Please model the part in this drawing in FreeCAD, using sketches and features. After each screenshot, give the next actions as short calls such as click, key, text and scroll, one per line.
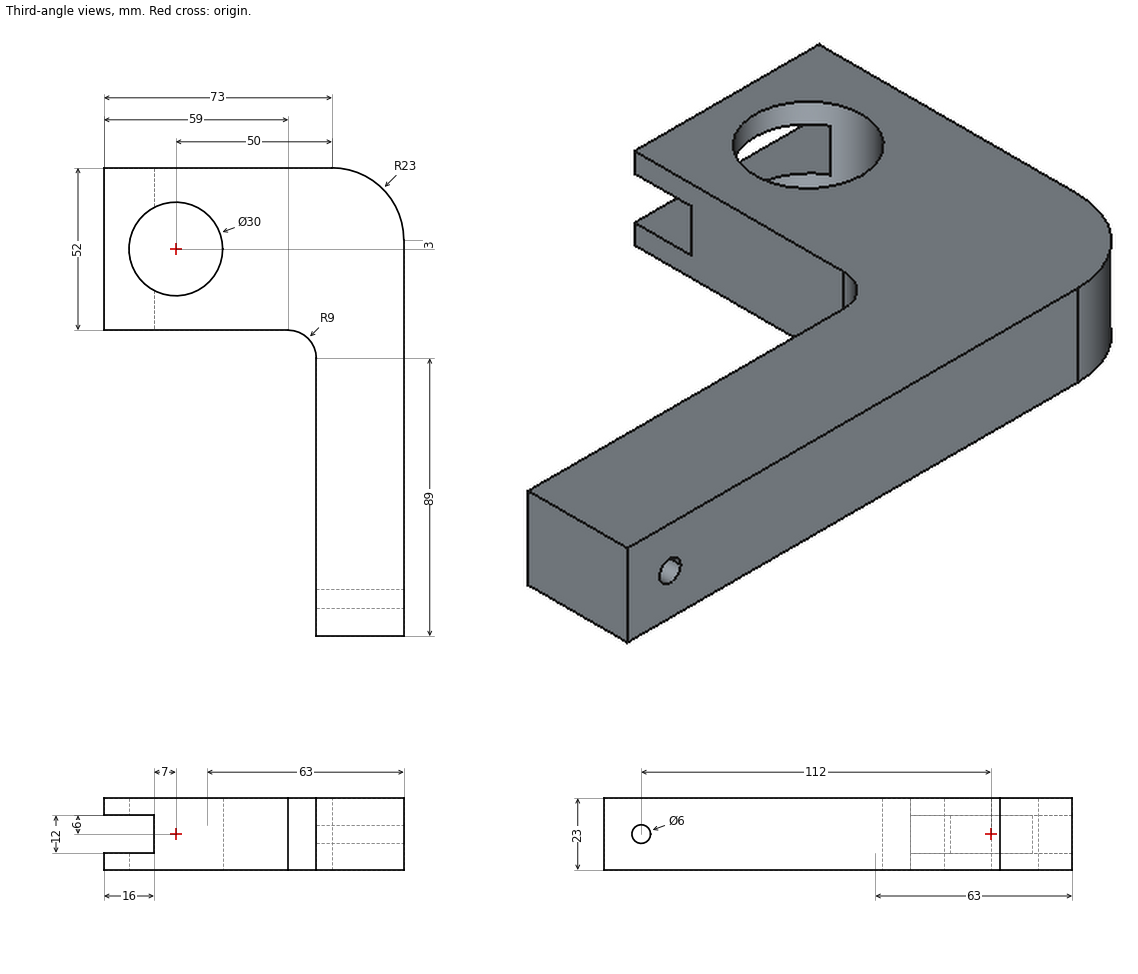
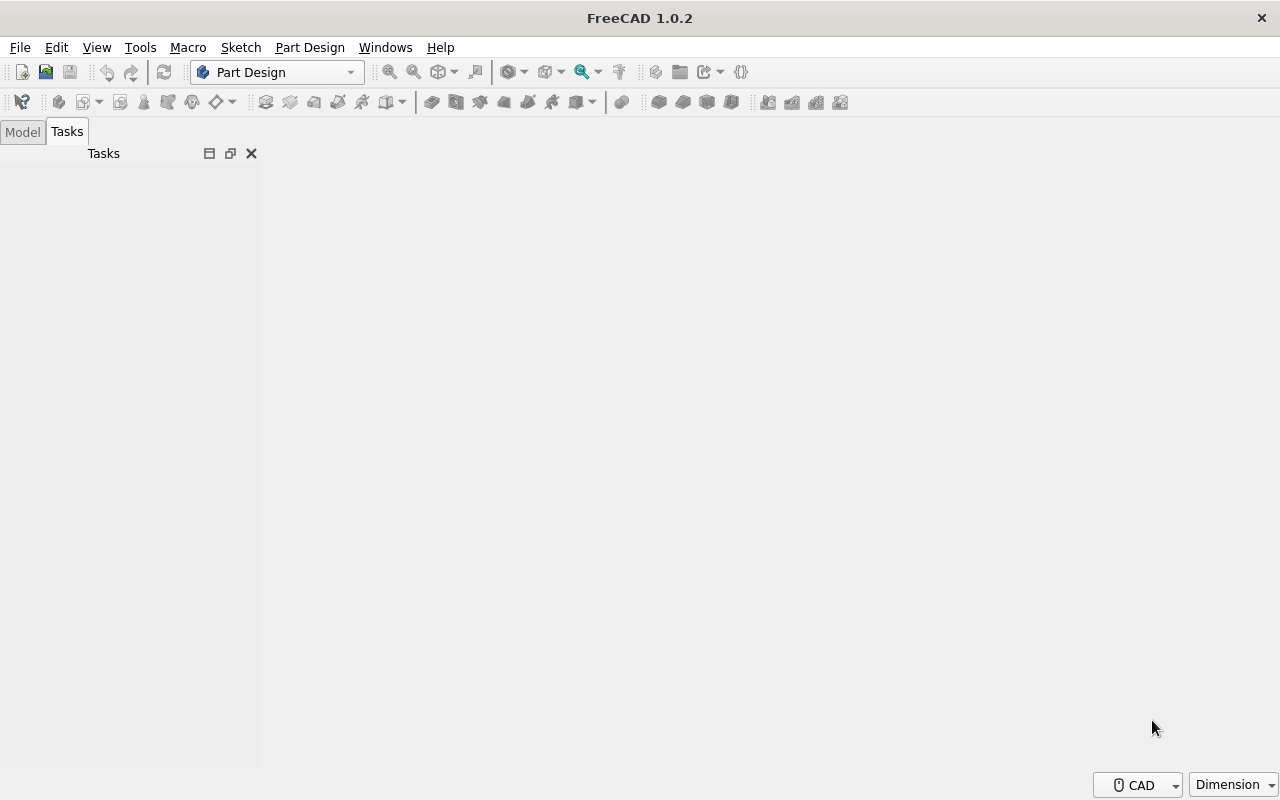
click(22, 72)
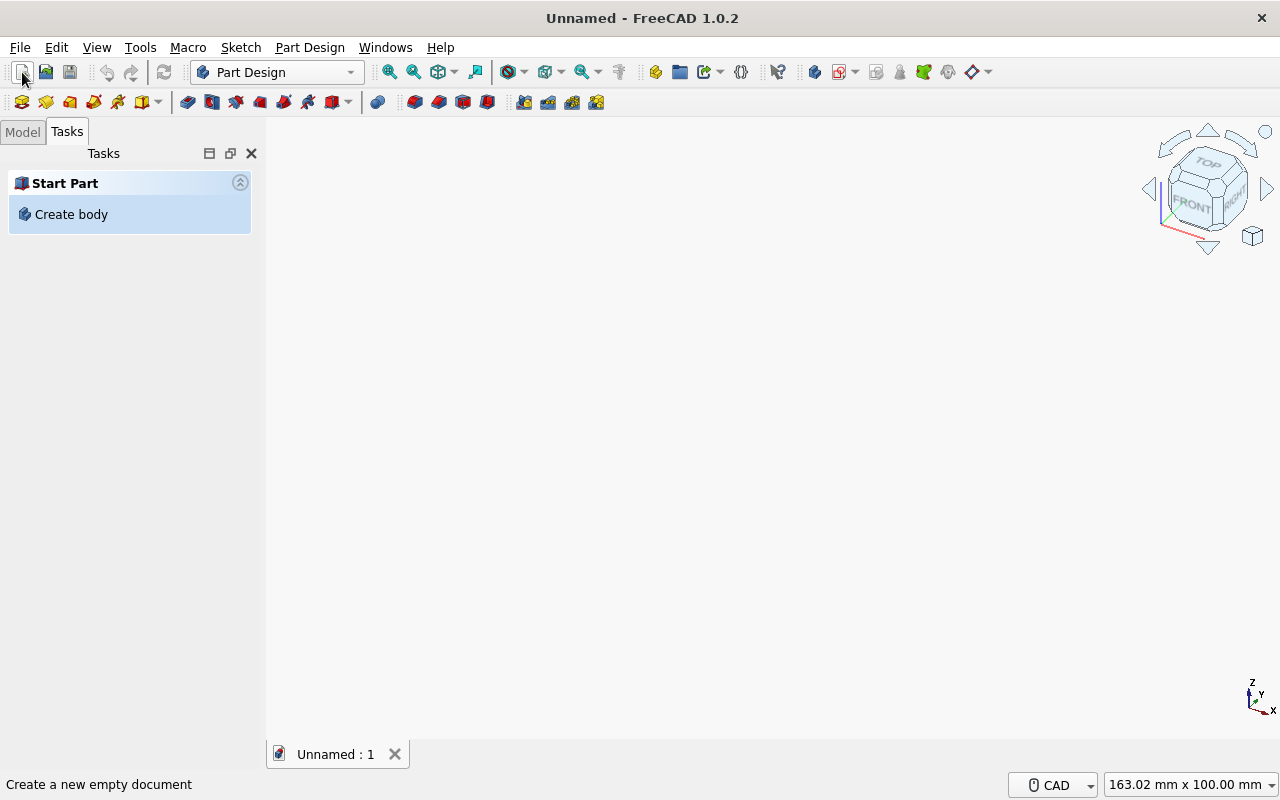
click(840, 72)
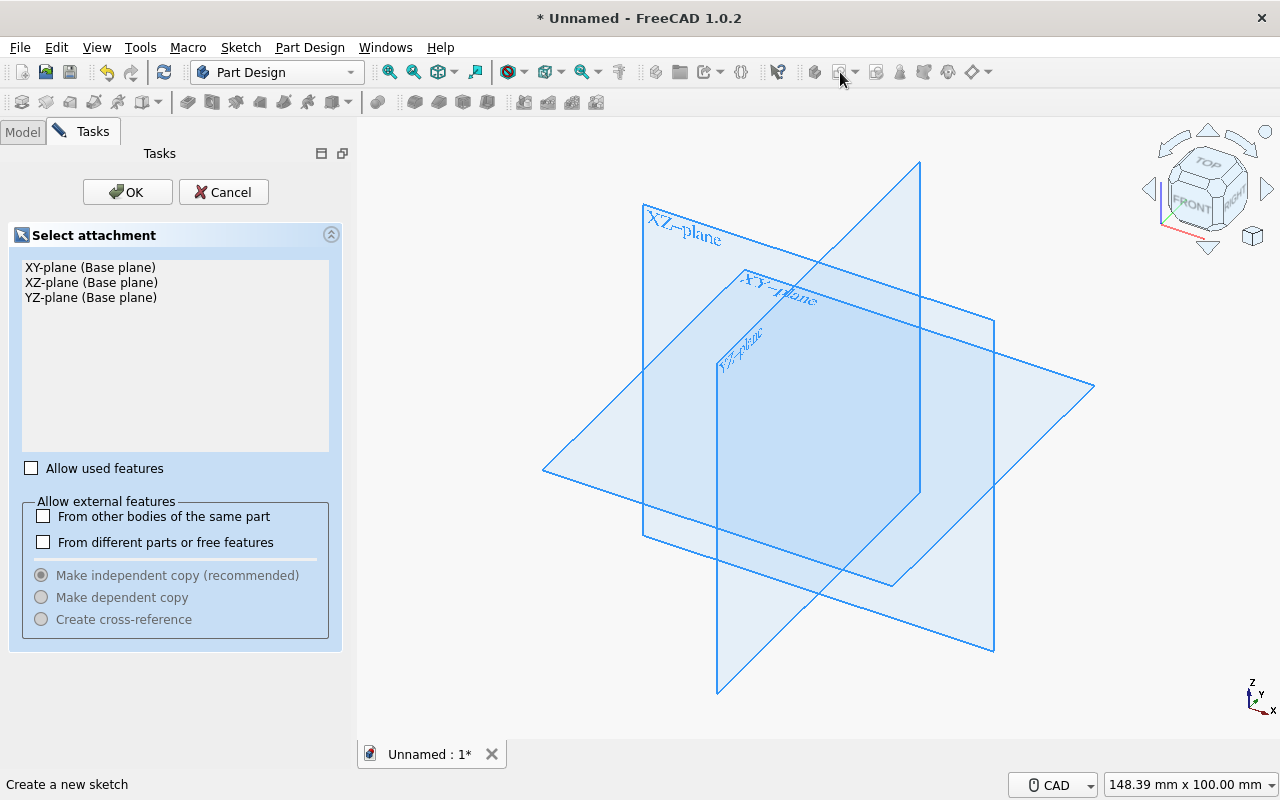
click(82, 268)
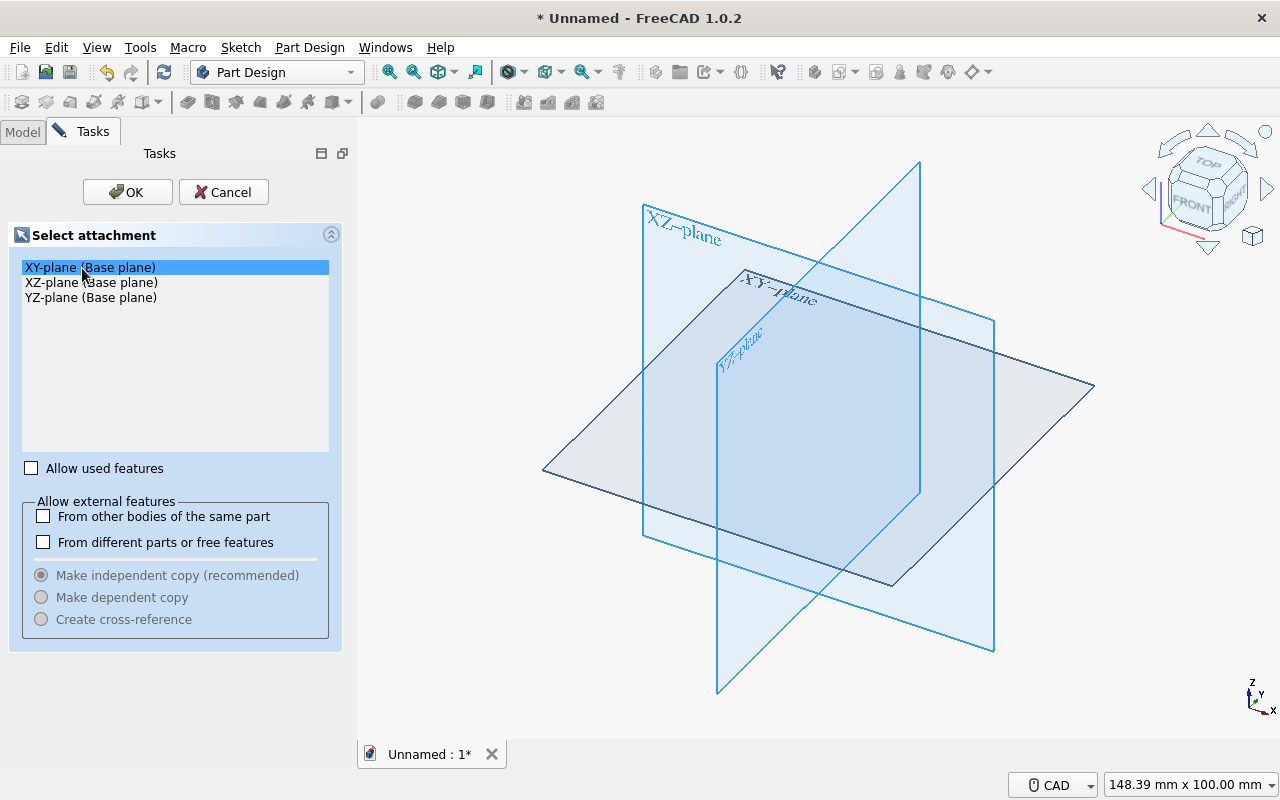
click(128, 192)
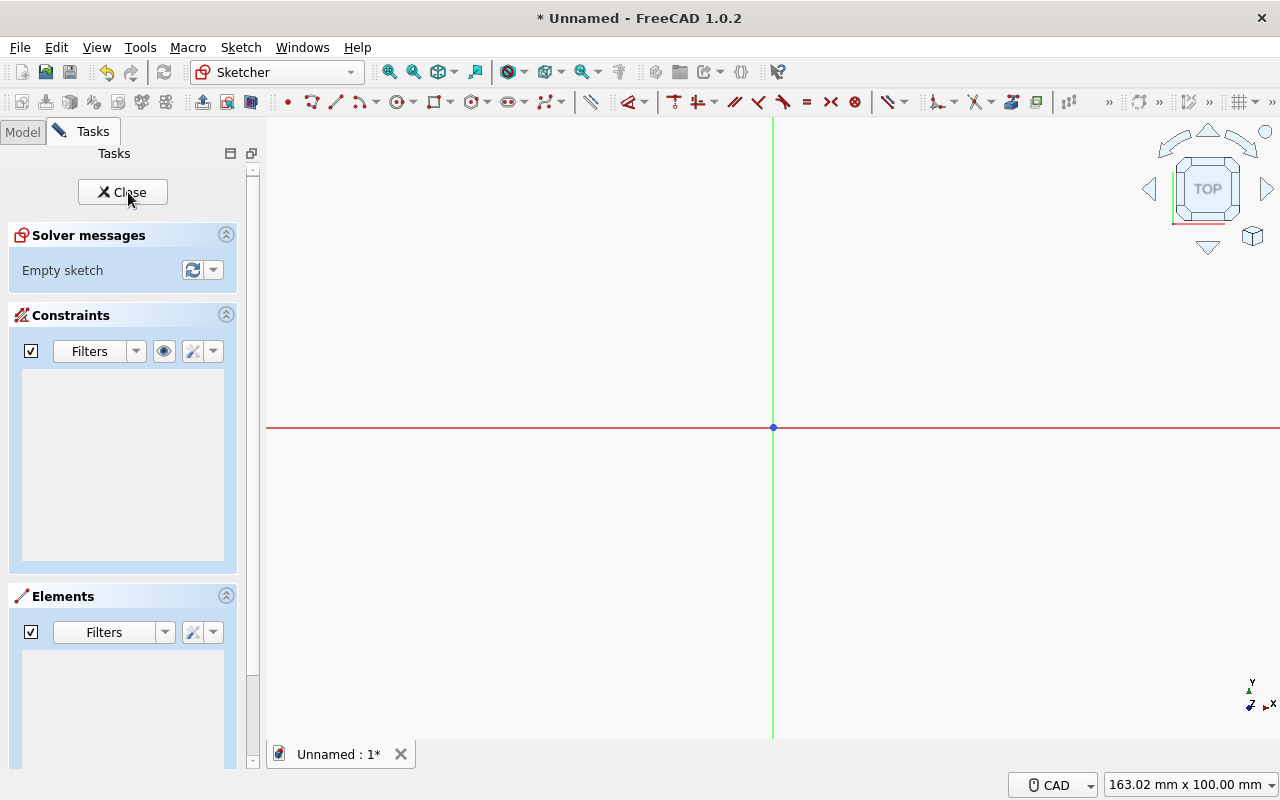
scroll(522, 179, down, 4)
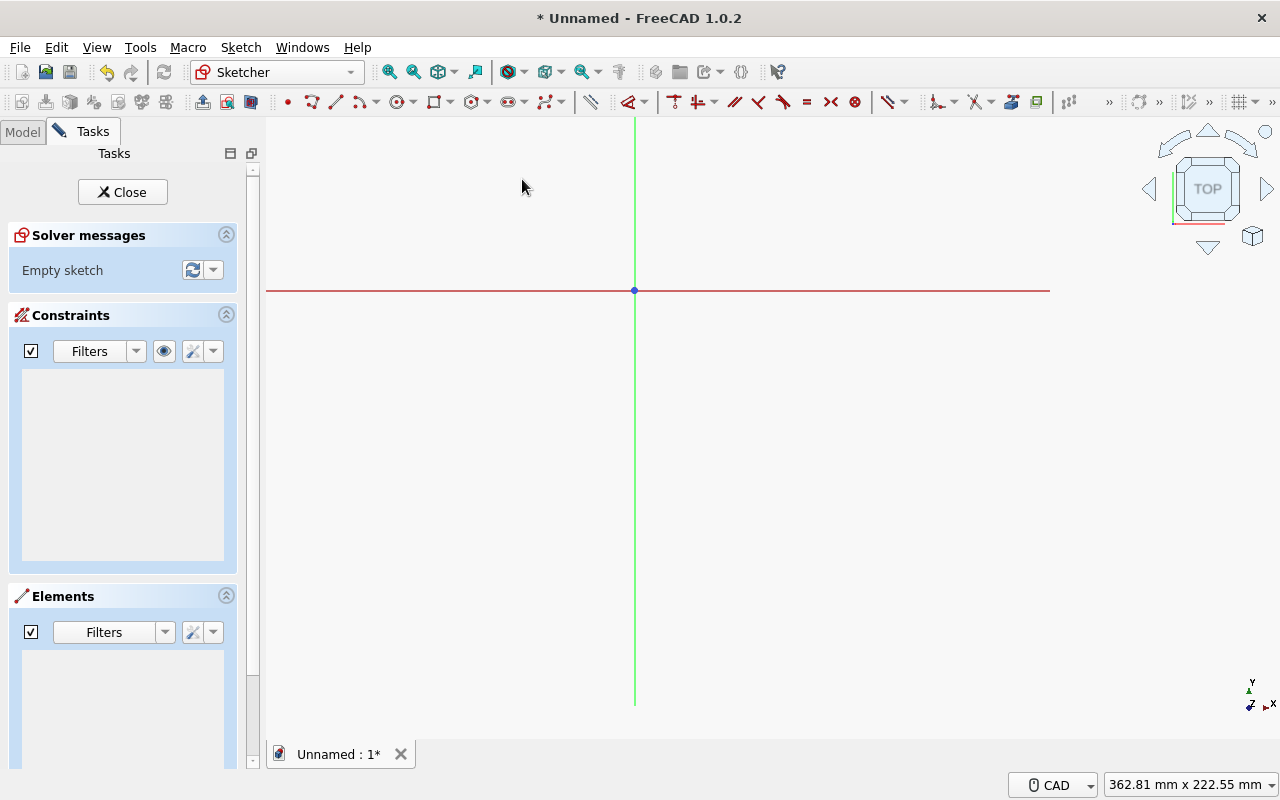
click(312, 102)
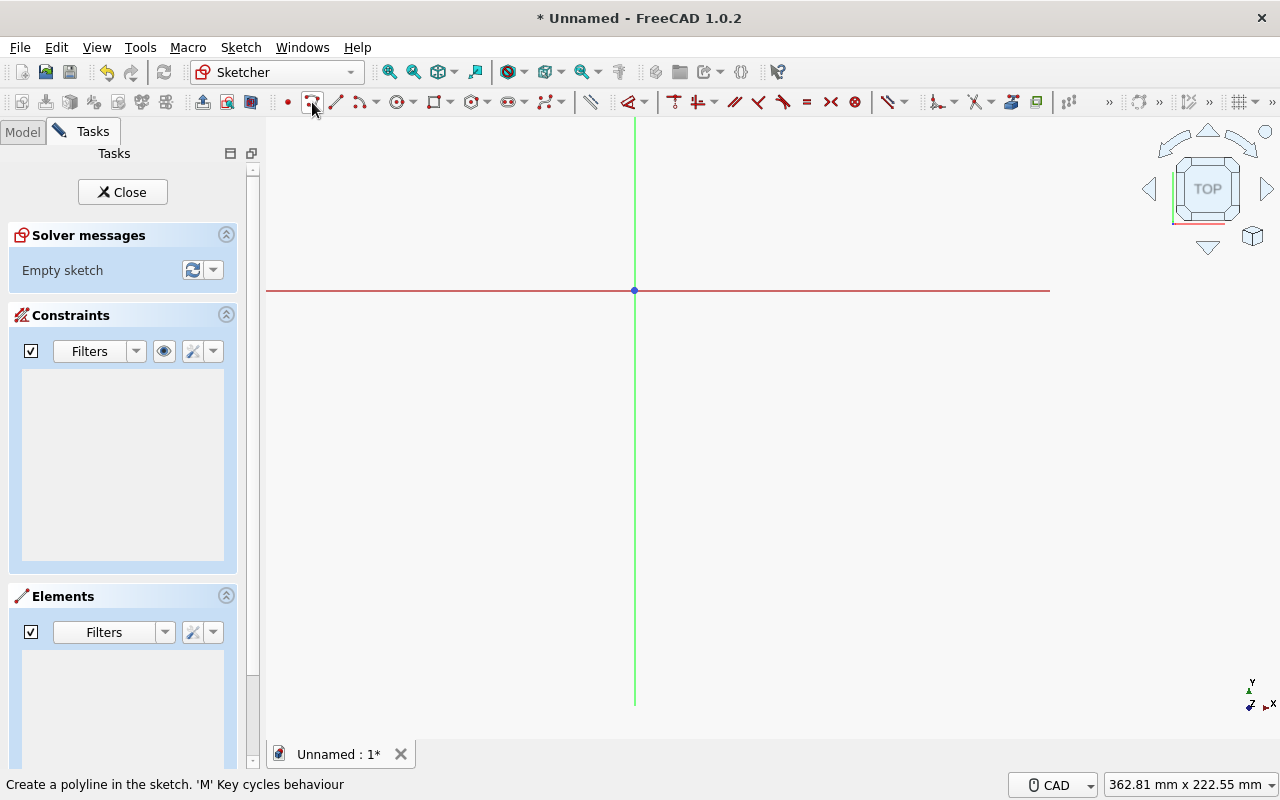
click(775, 218)
click(571, 218)
click(571, 364)
click(736, 364)
right_click(736, 364)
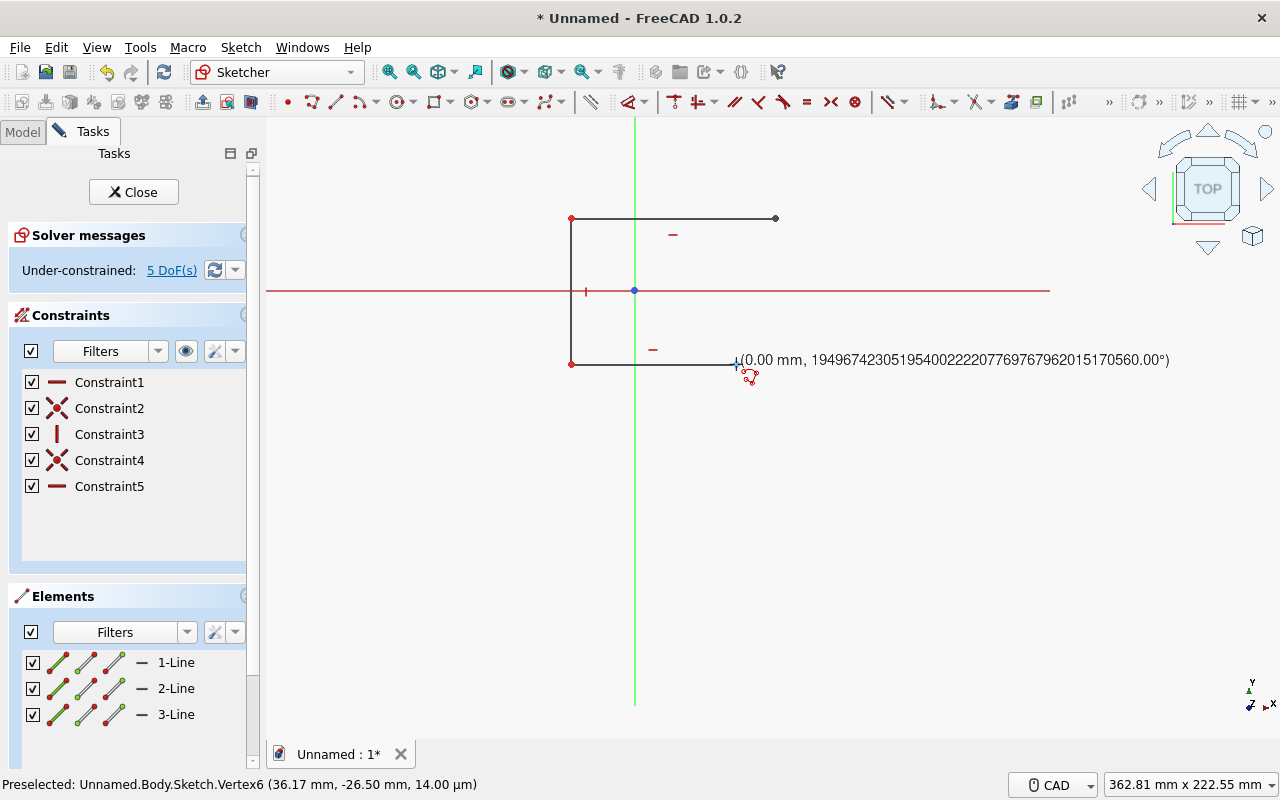
click(761, 389)
click(761, 637)
click(839, 637)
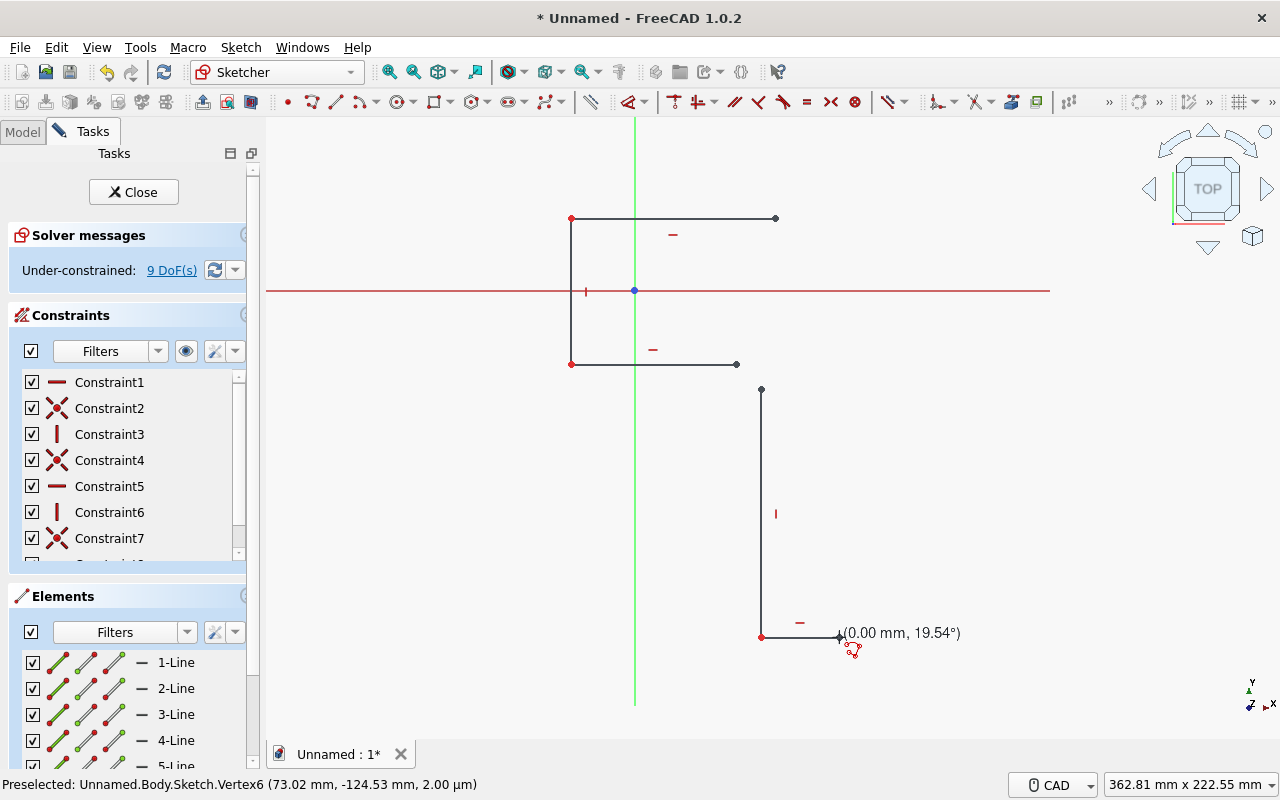
scroll(839, 283, up, 4)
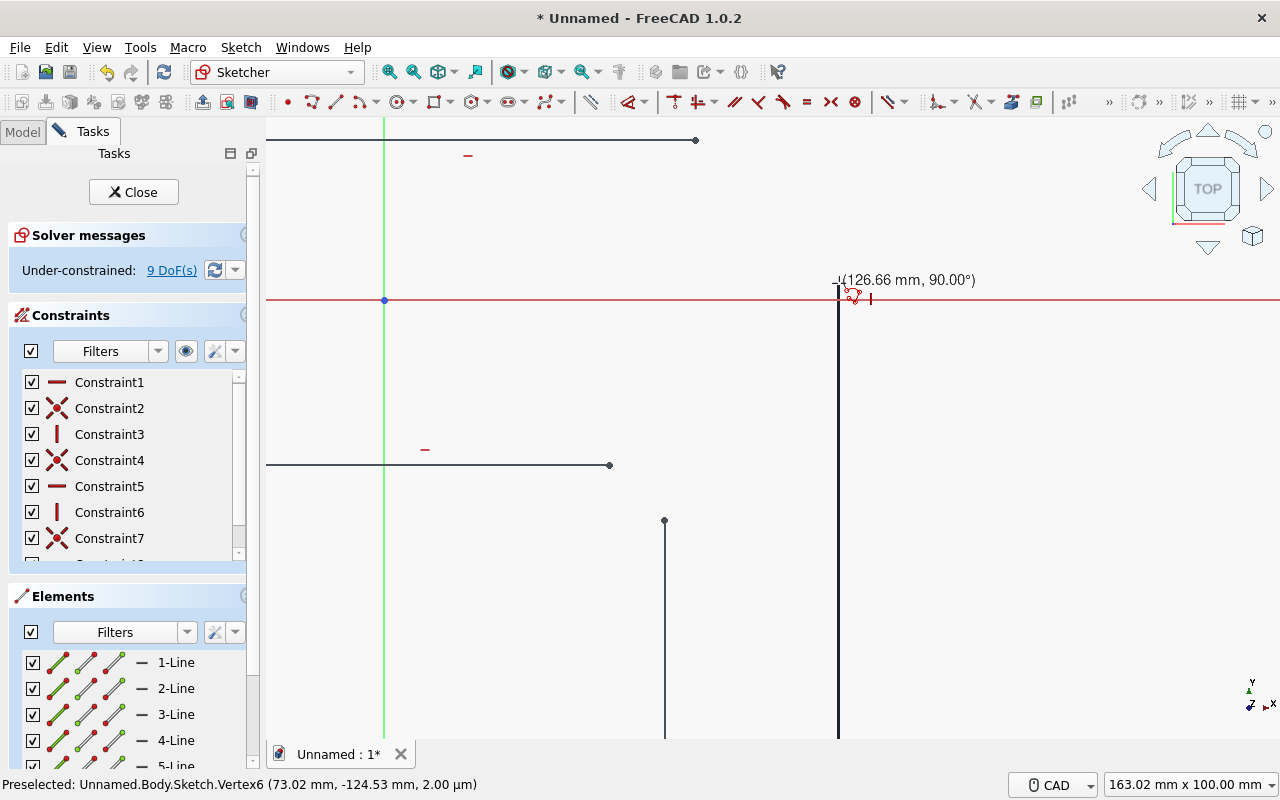
click(838, 282)
right_click(838, 282)